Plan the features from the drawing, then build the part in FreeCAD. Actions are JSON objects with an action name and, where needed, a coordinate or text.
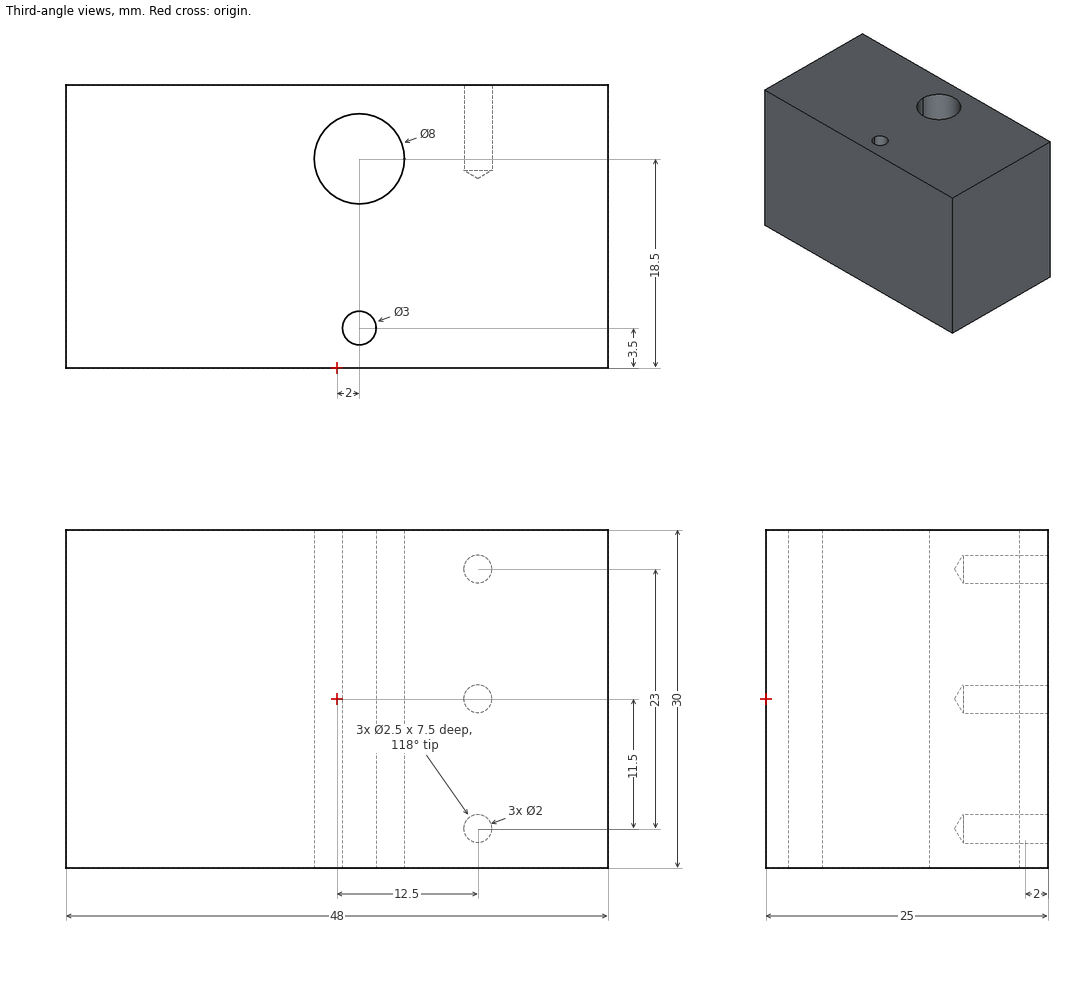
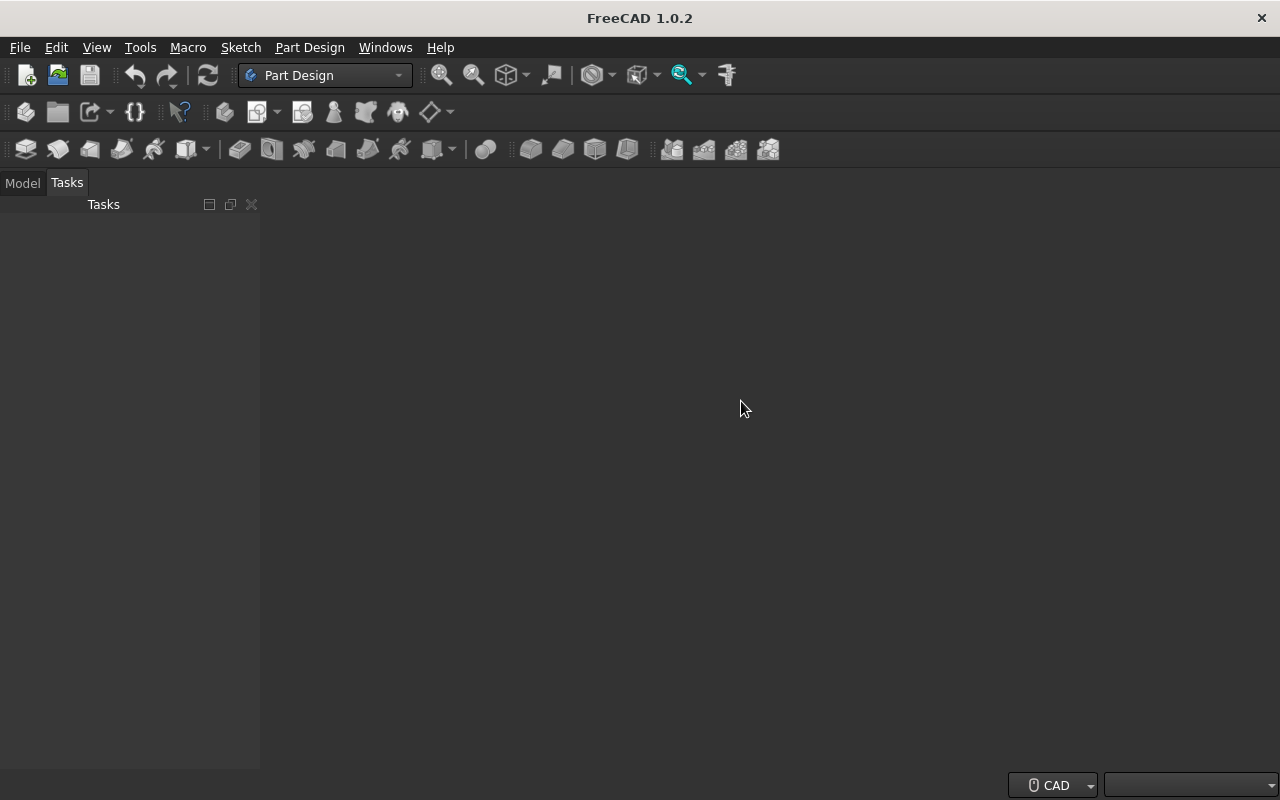
{"action": "key", "text": "ctrl+n"}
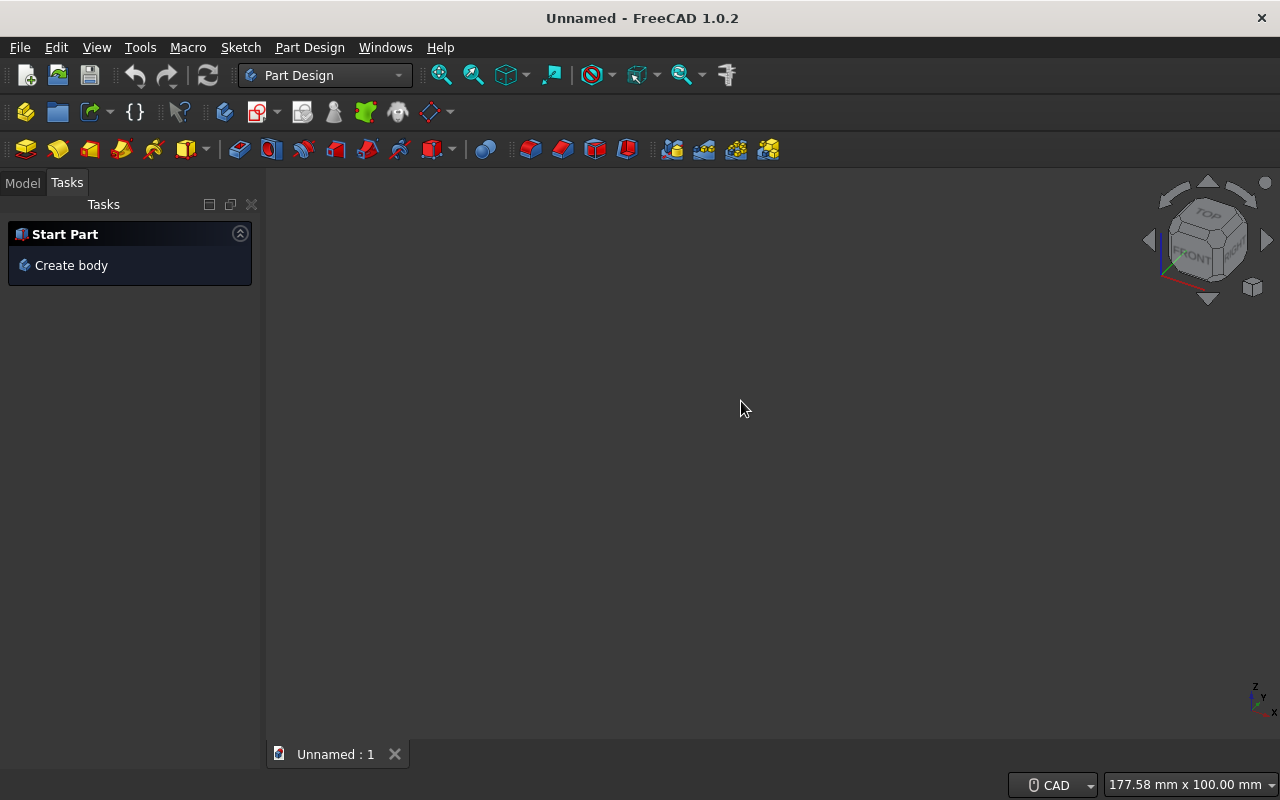
{"action": "left_click", "coordinate": [258, 112]}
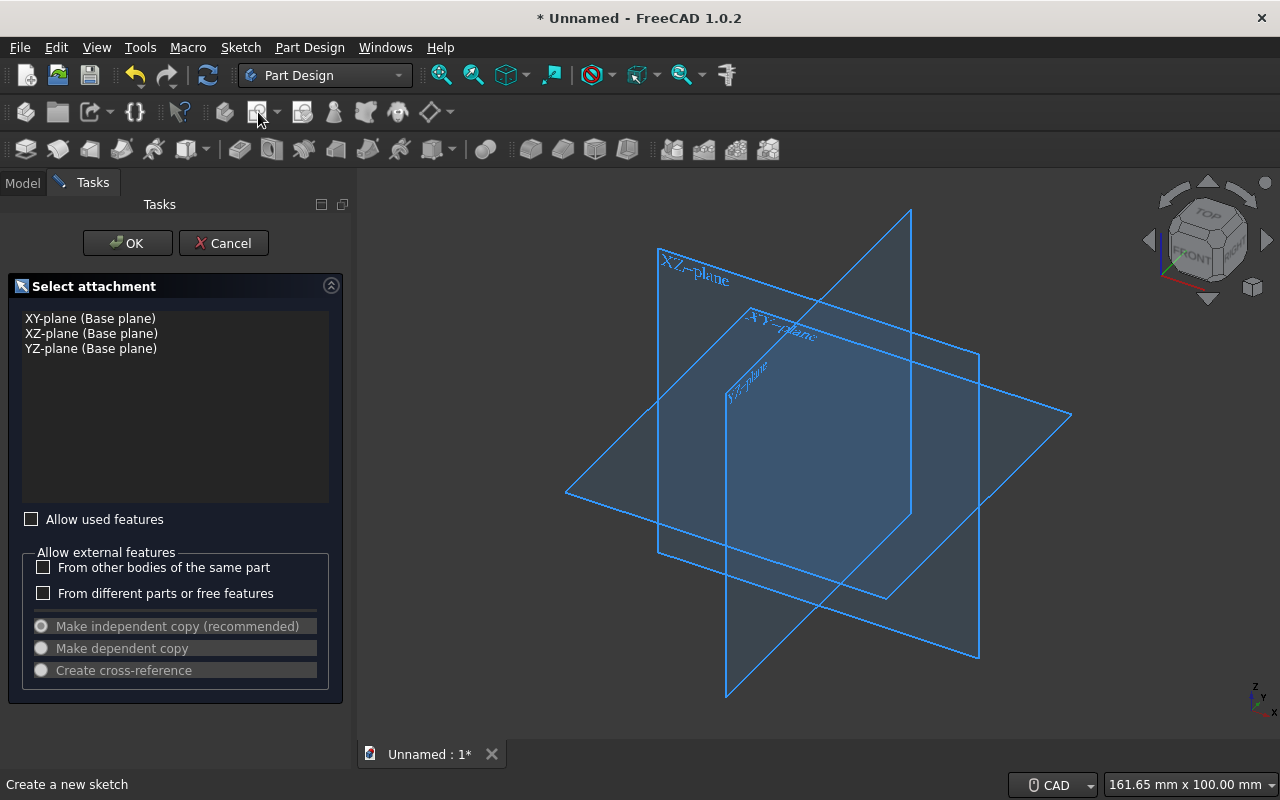
{"action": "left_click", "coordinate": [82, 334]}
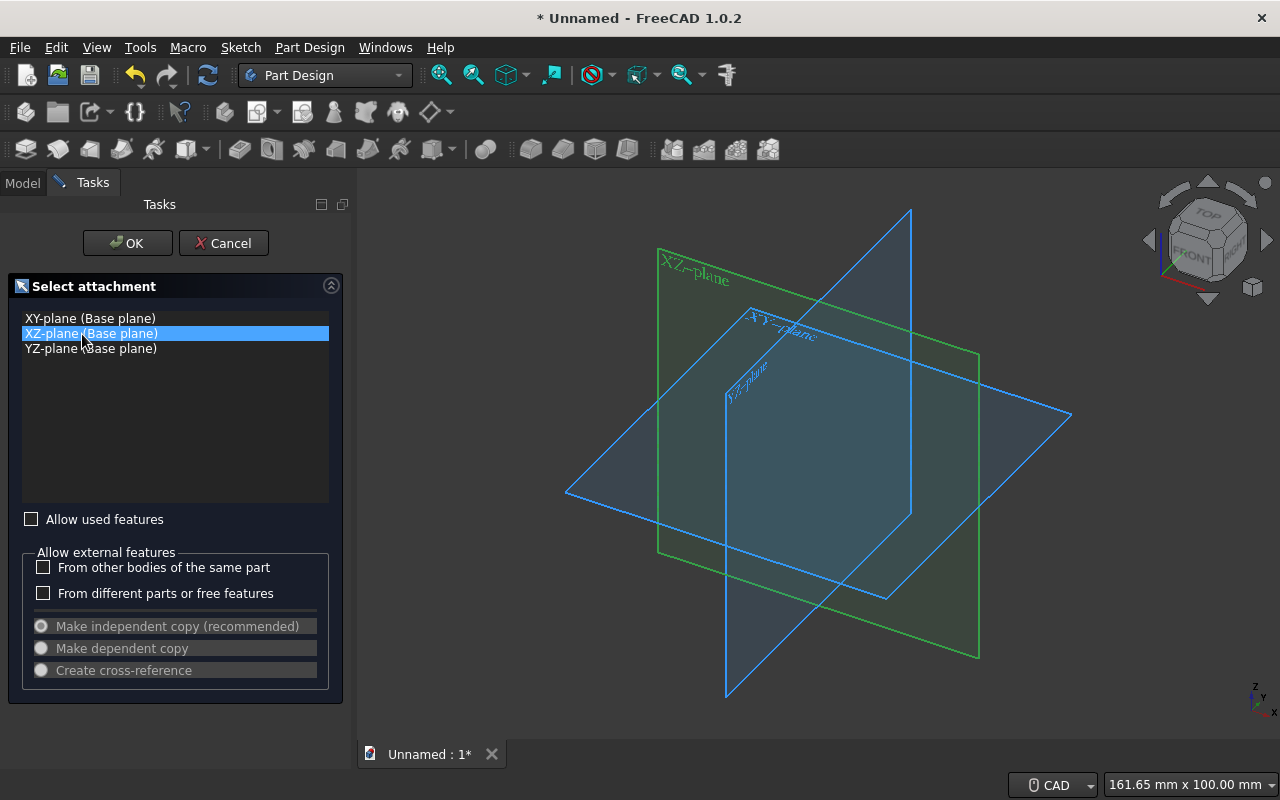
{"action": "left_click", "coordinate": [128, 243]}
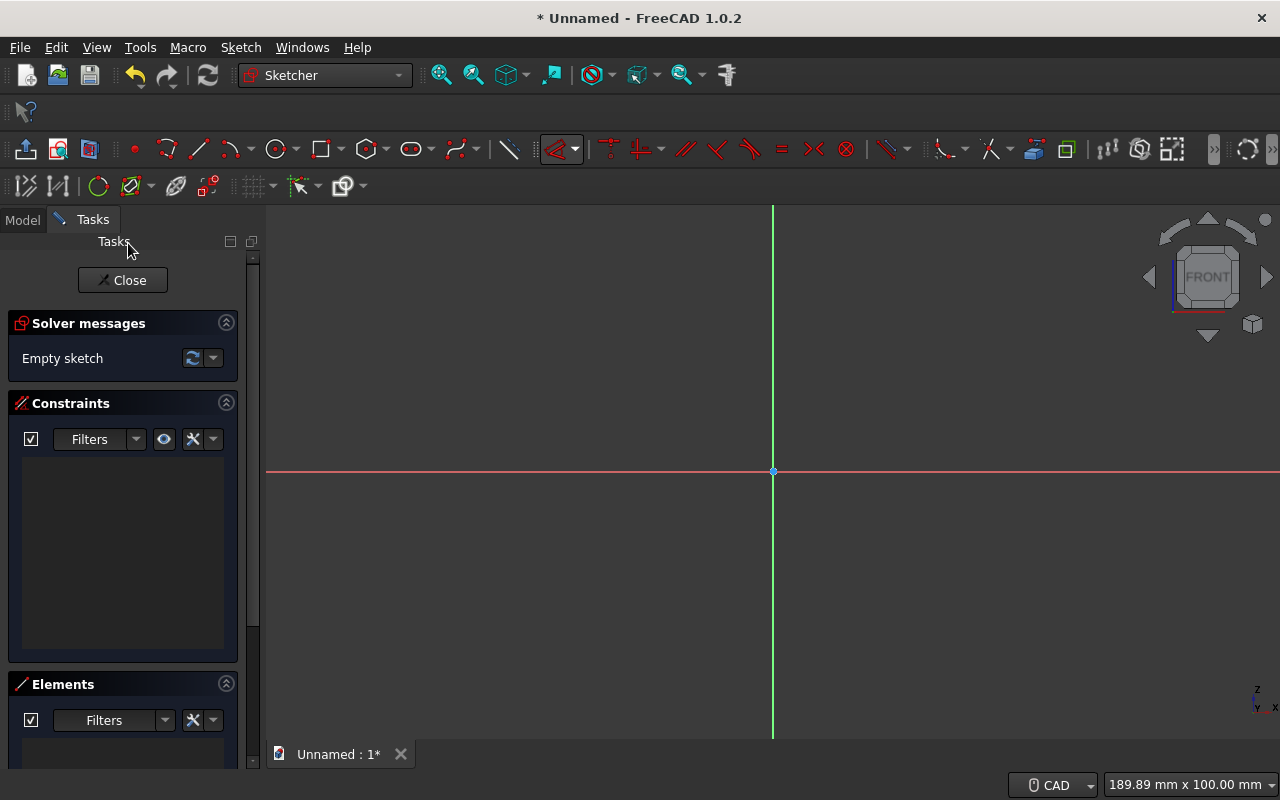
{"action": "scroll", "coordinate": [829, 472], "scroll_direction": "up", "scroll_amount": 4}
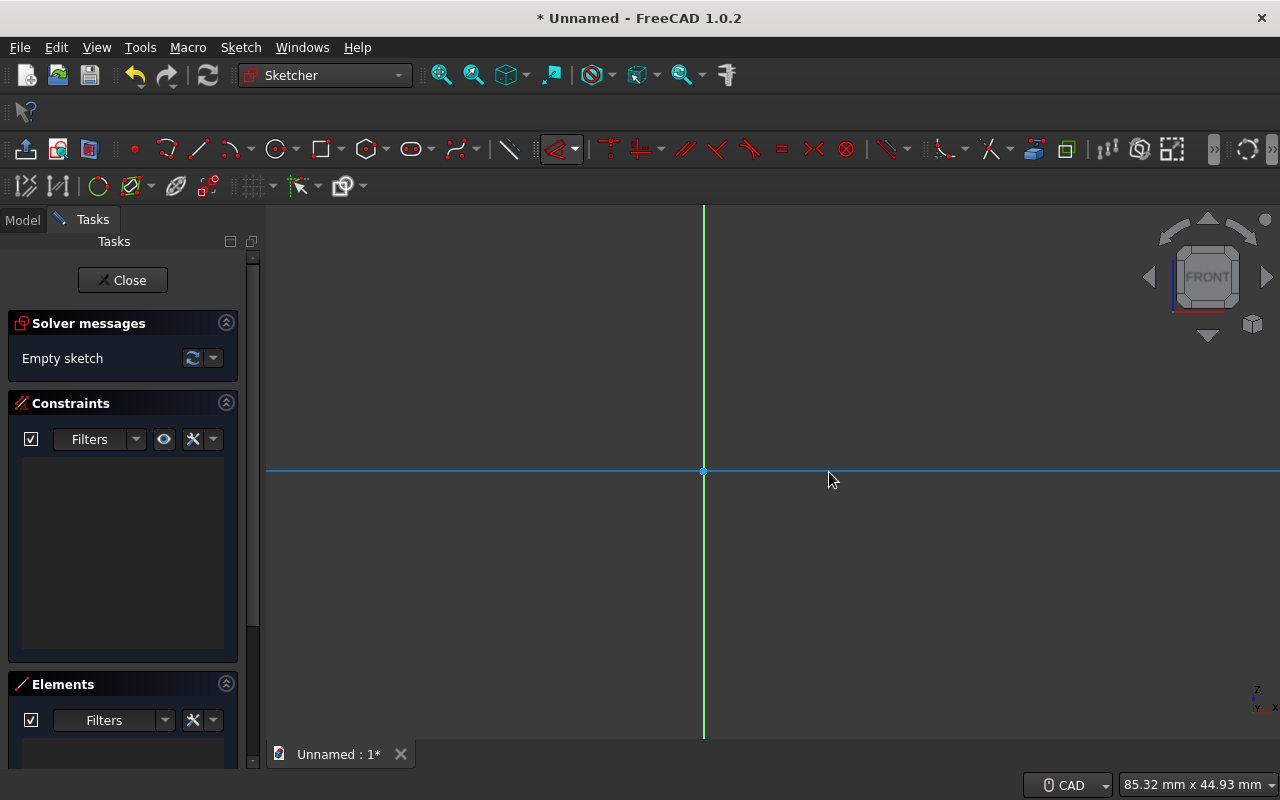
{"action": "left_click", "coordinate": [344, 150]}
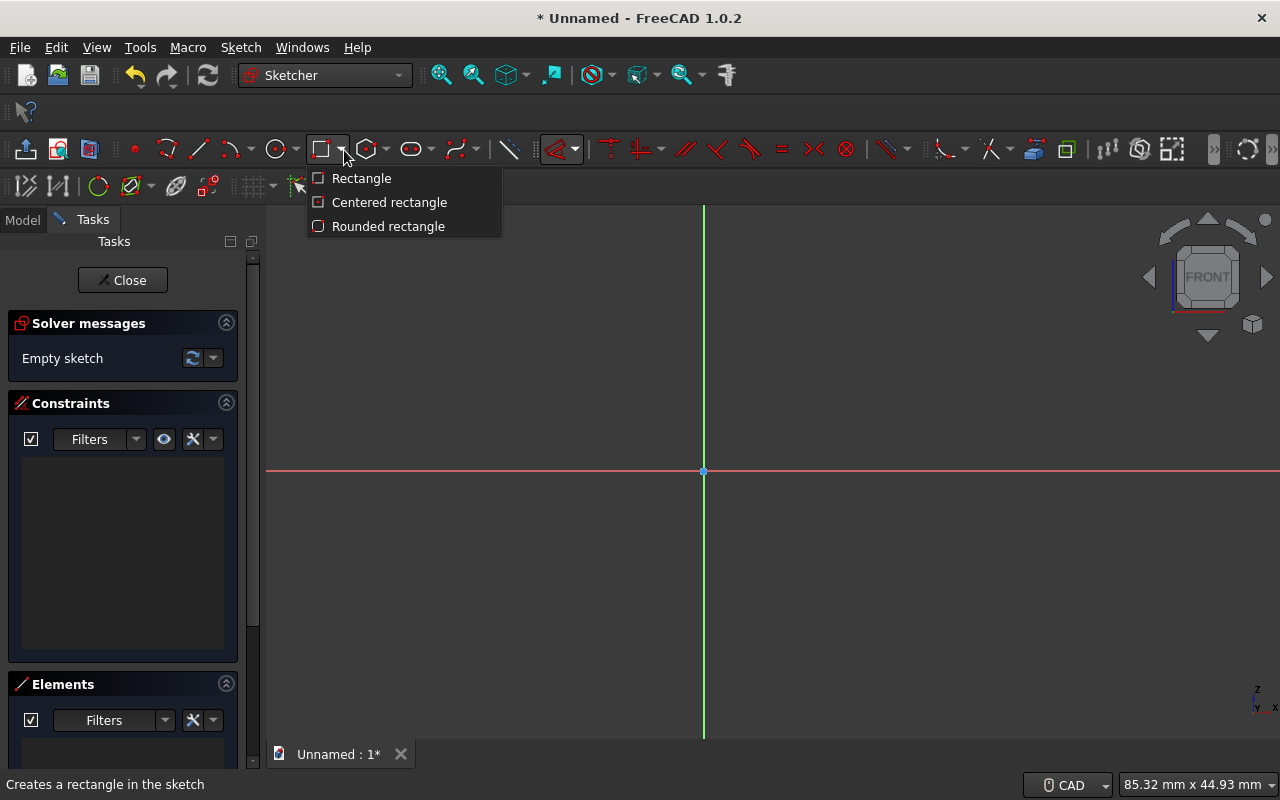
{"action": "left_click", "coordinate": [404, 202]}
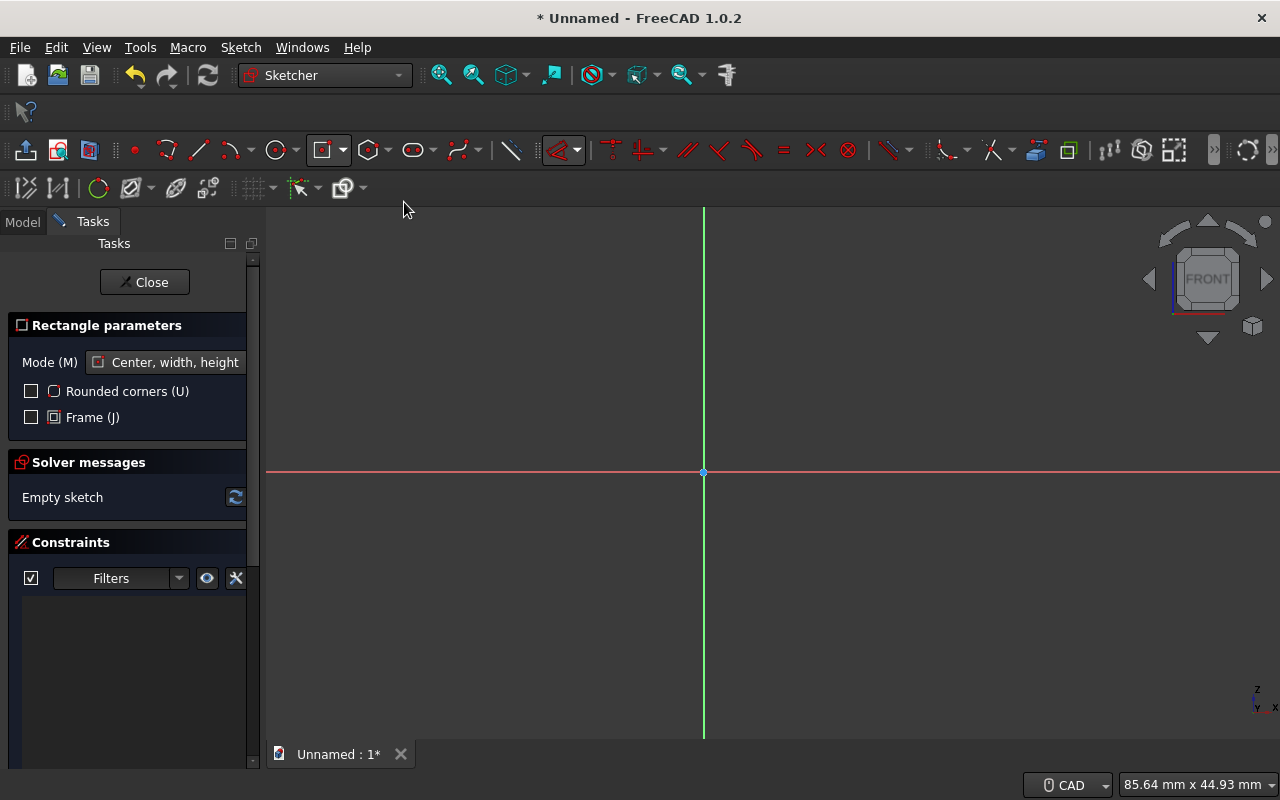
{"action": "left_click", "coordinate": [704, 472]}
{"action": "left_click", "coordinate": [988, 295]}
{"action": "key", "text": "Escape"}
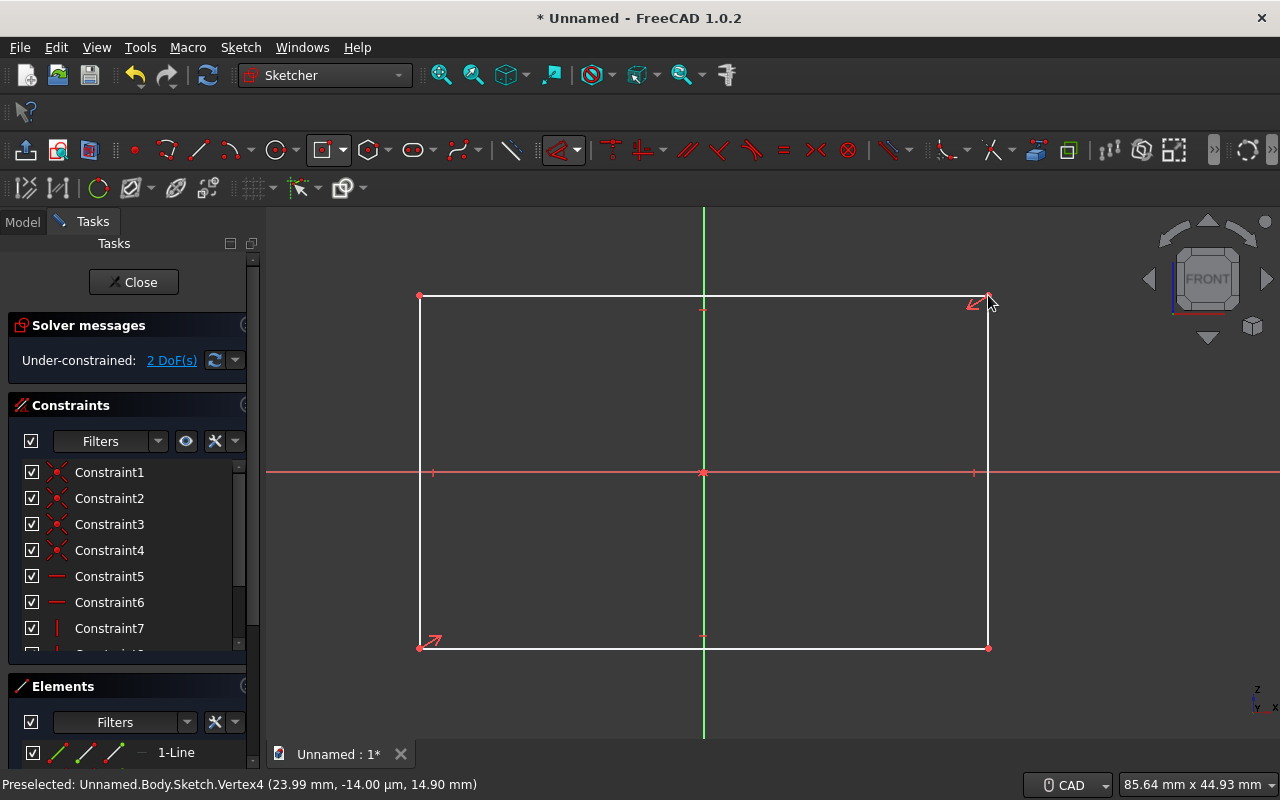
{"action": "key", "text": "d"}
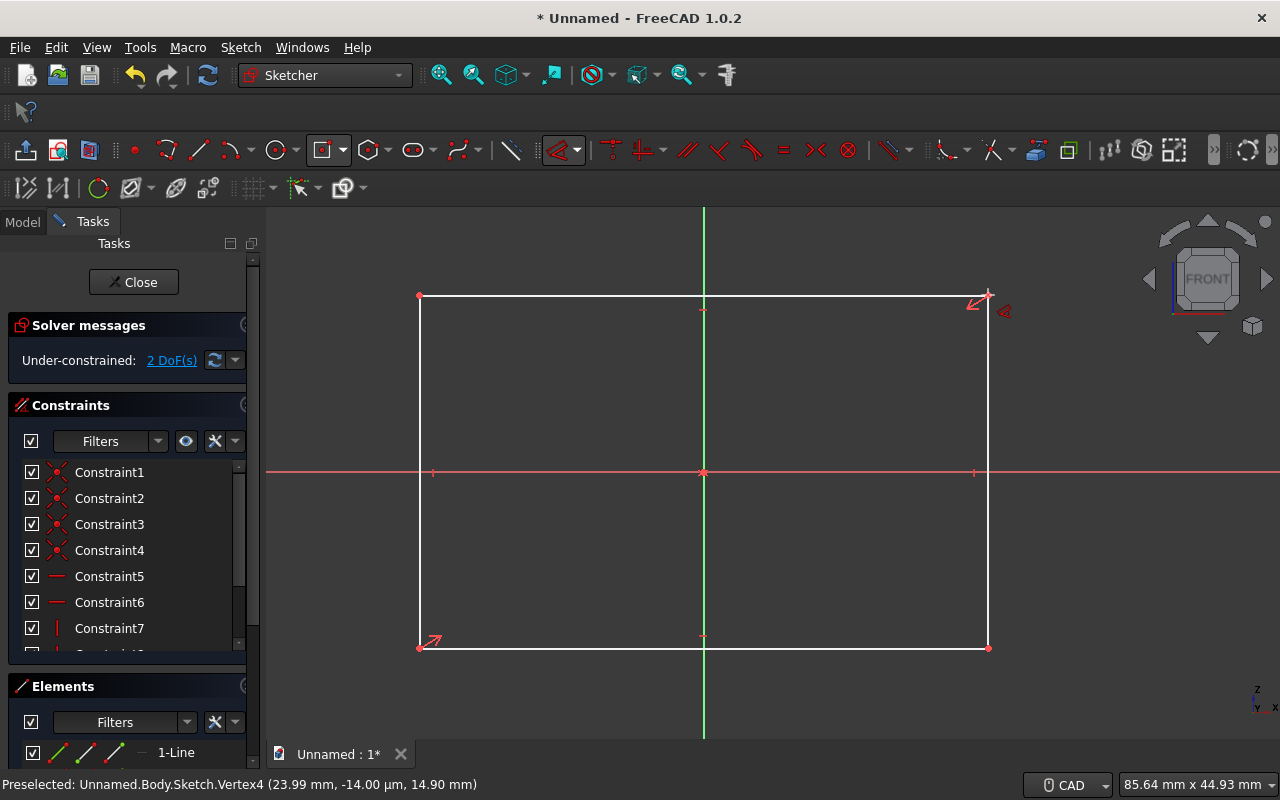
{"action": "left_click", "coordinate": [590, 649]}
{"action": "left_click", "coordinate": [573, 683]}